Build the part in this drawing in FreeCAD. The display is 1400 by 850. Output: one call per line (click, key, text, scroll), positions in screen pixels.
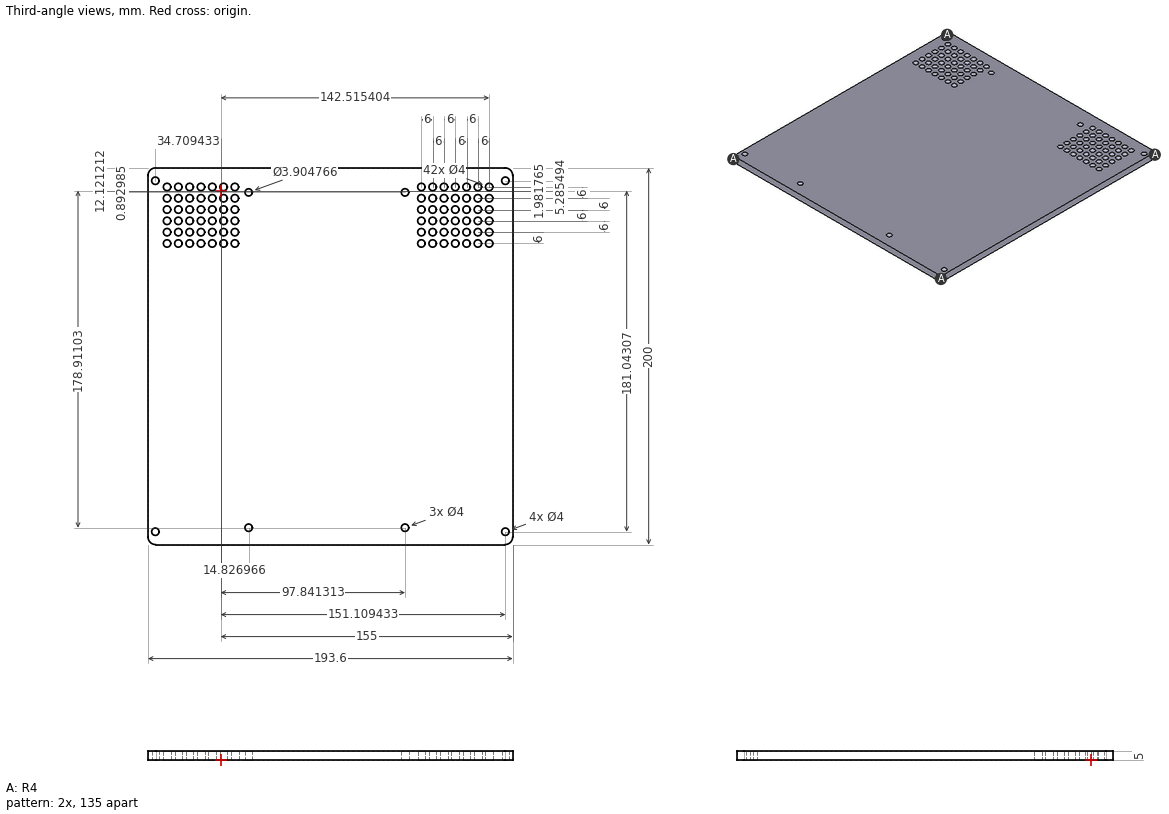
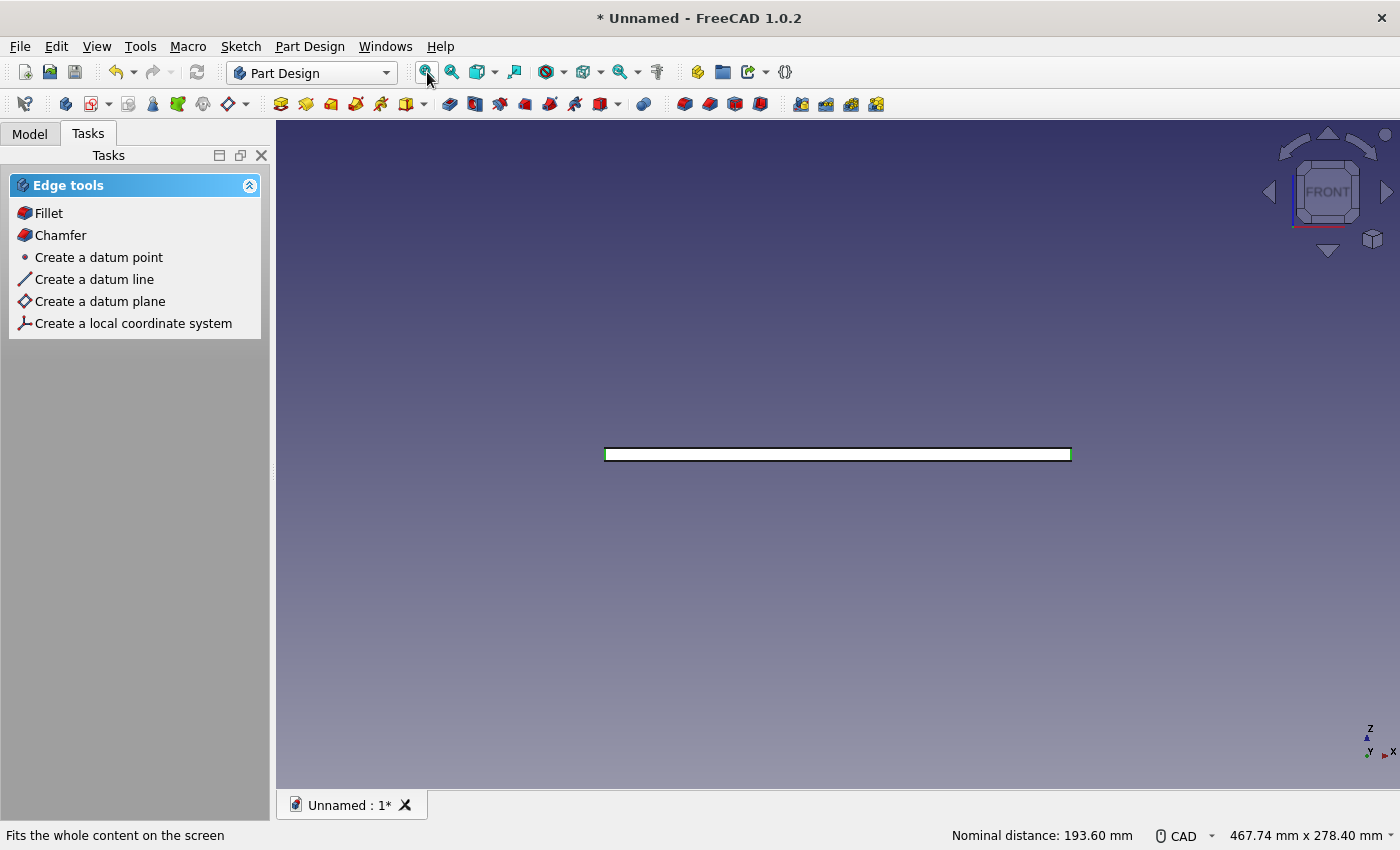
key(3)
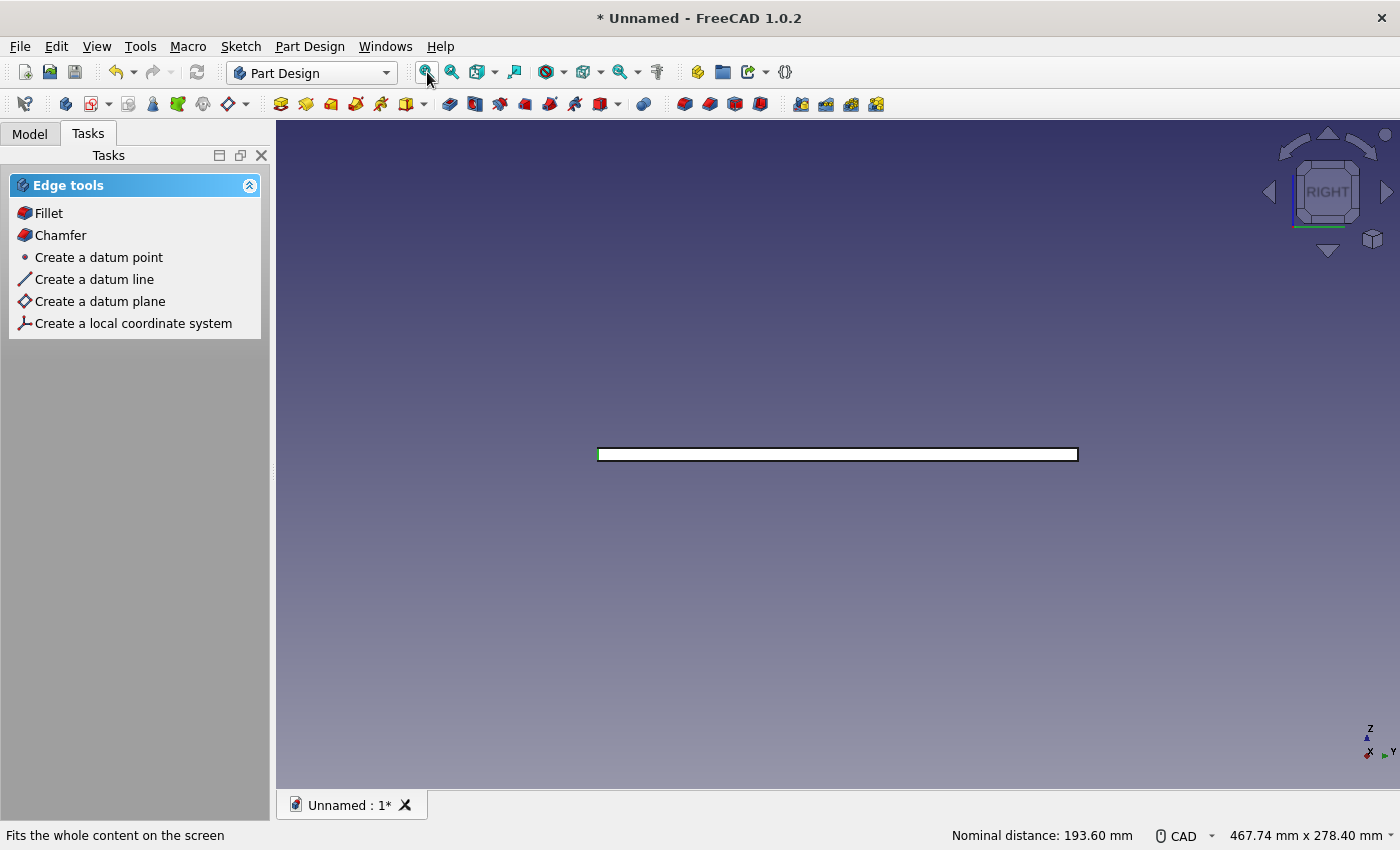
click(427, 72)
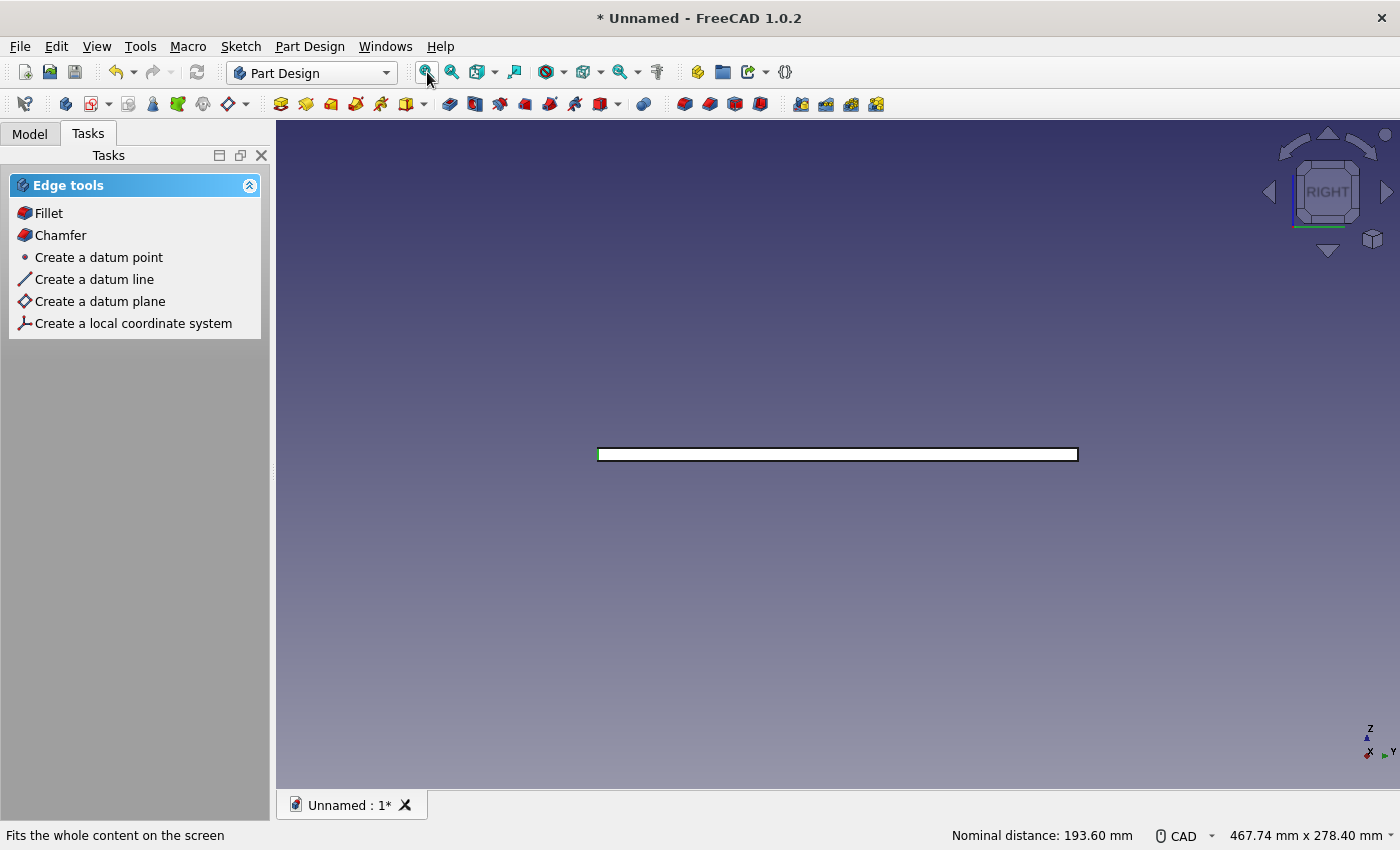
scroll(1078, 453, up, 7)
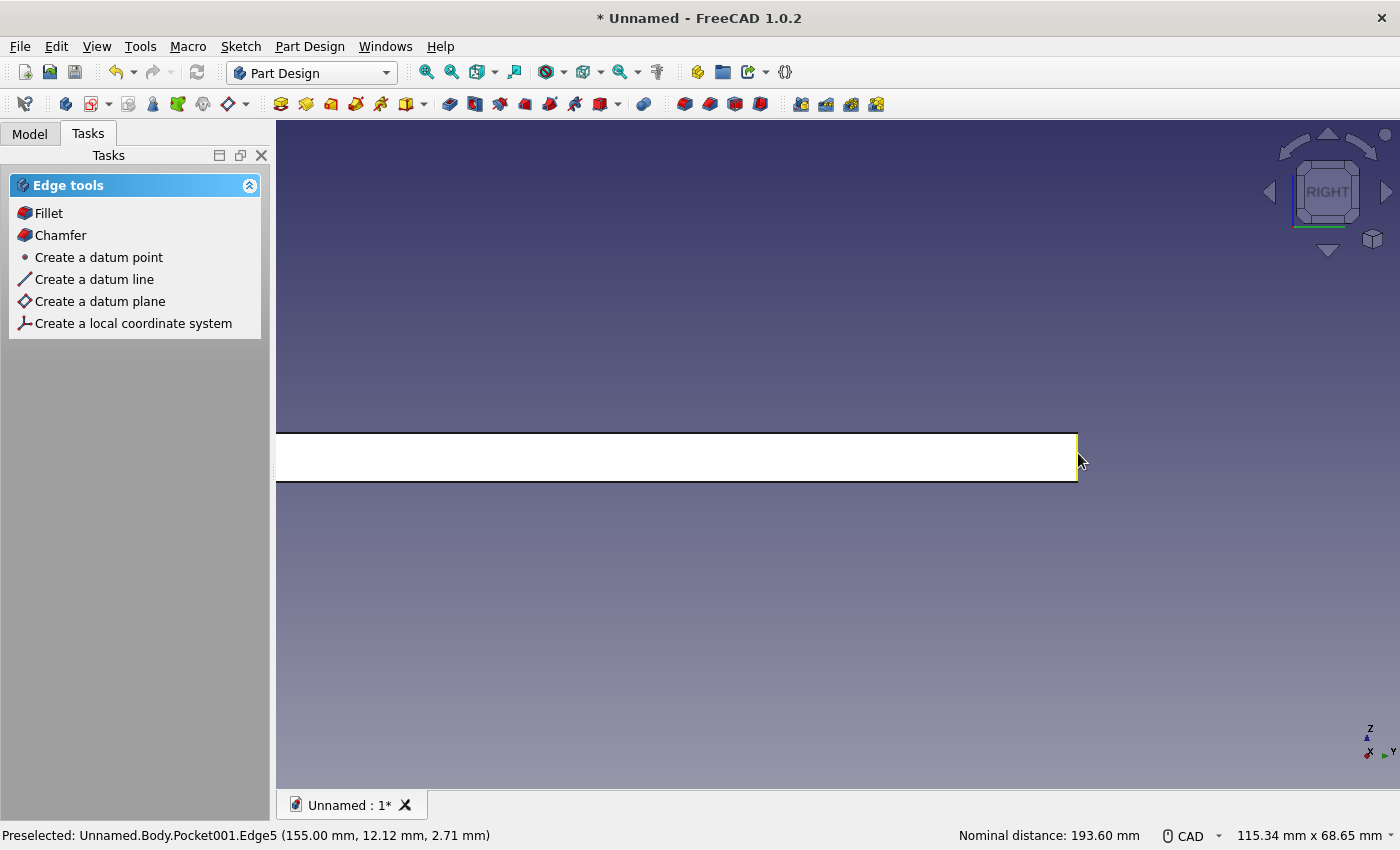
click(1077, 457, ctrl)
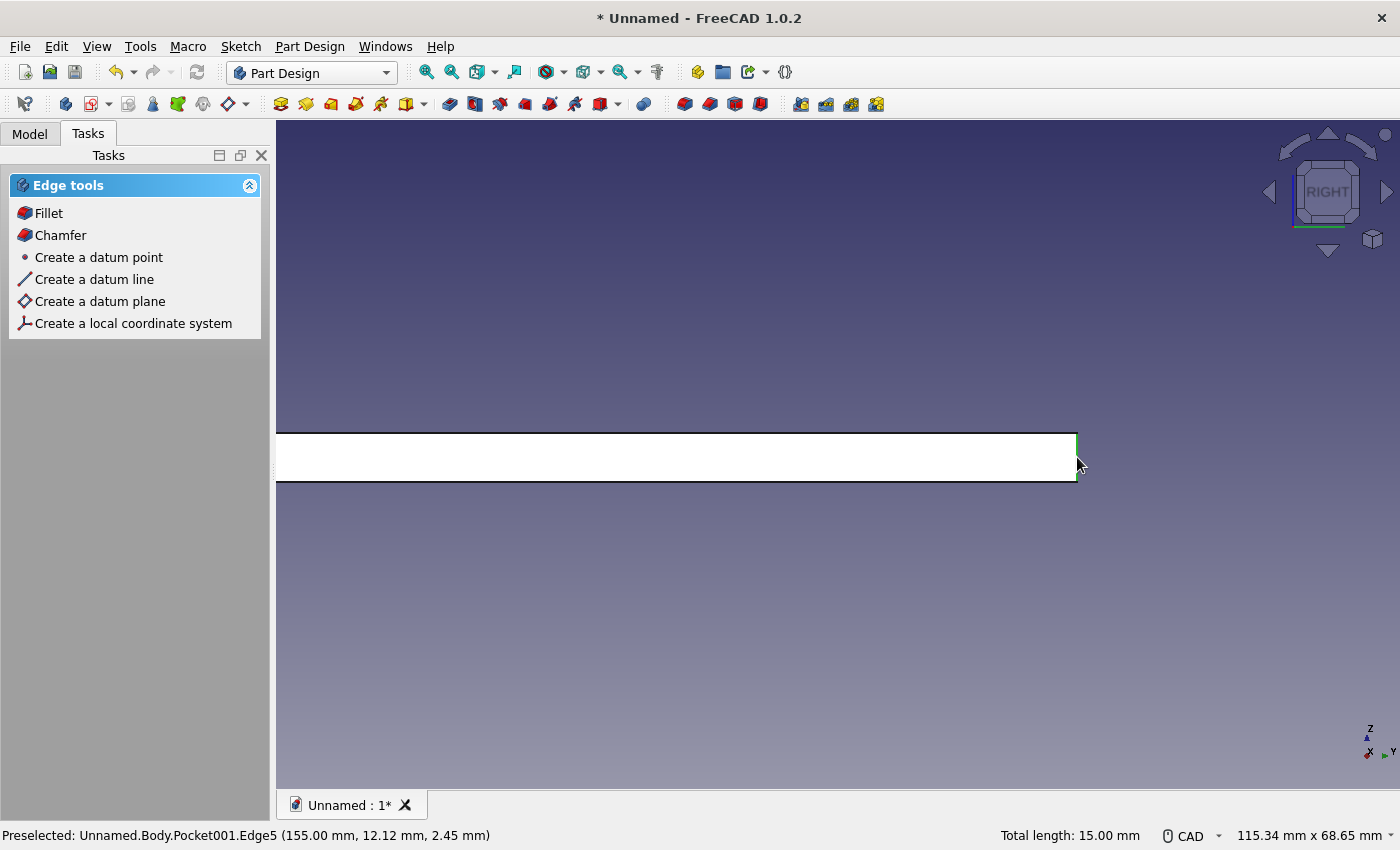
click(427, 72)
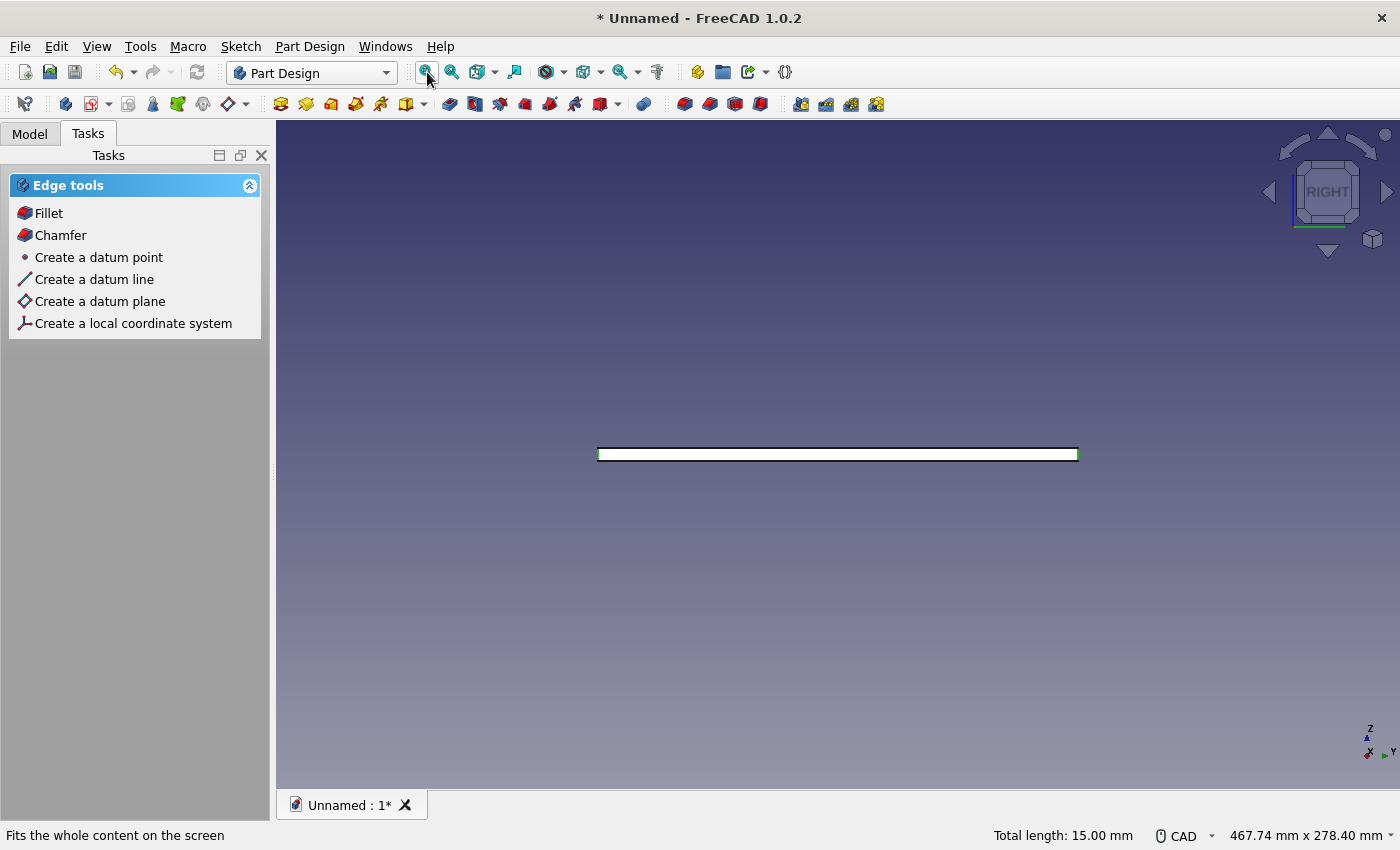
key(5)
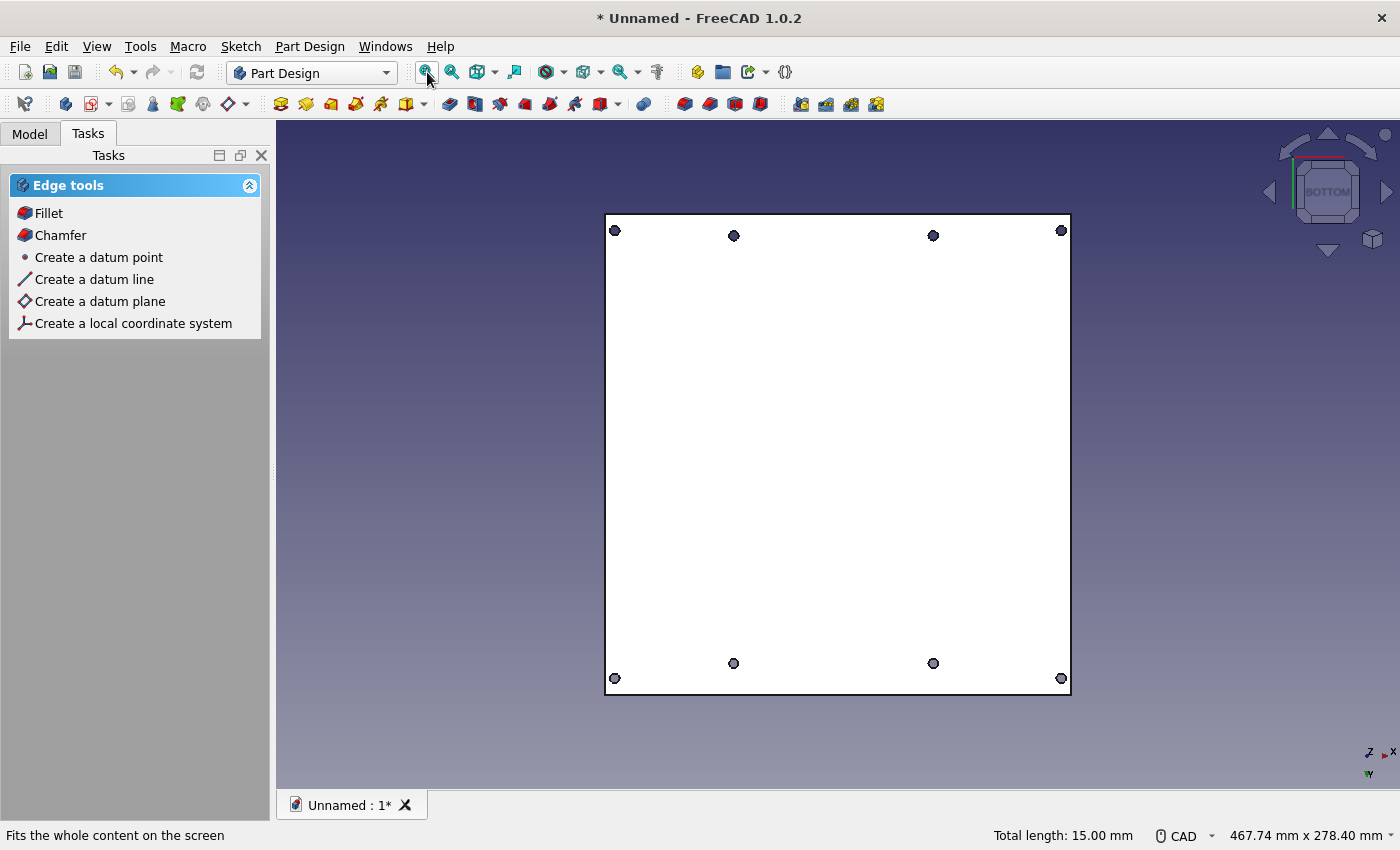
scroll(605, 694, up, 7)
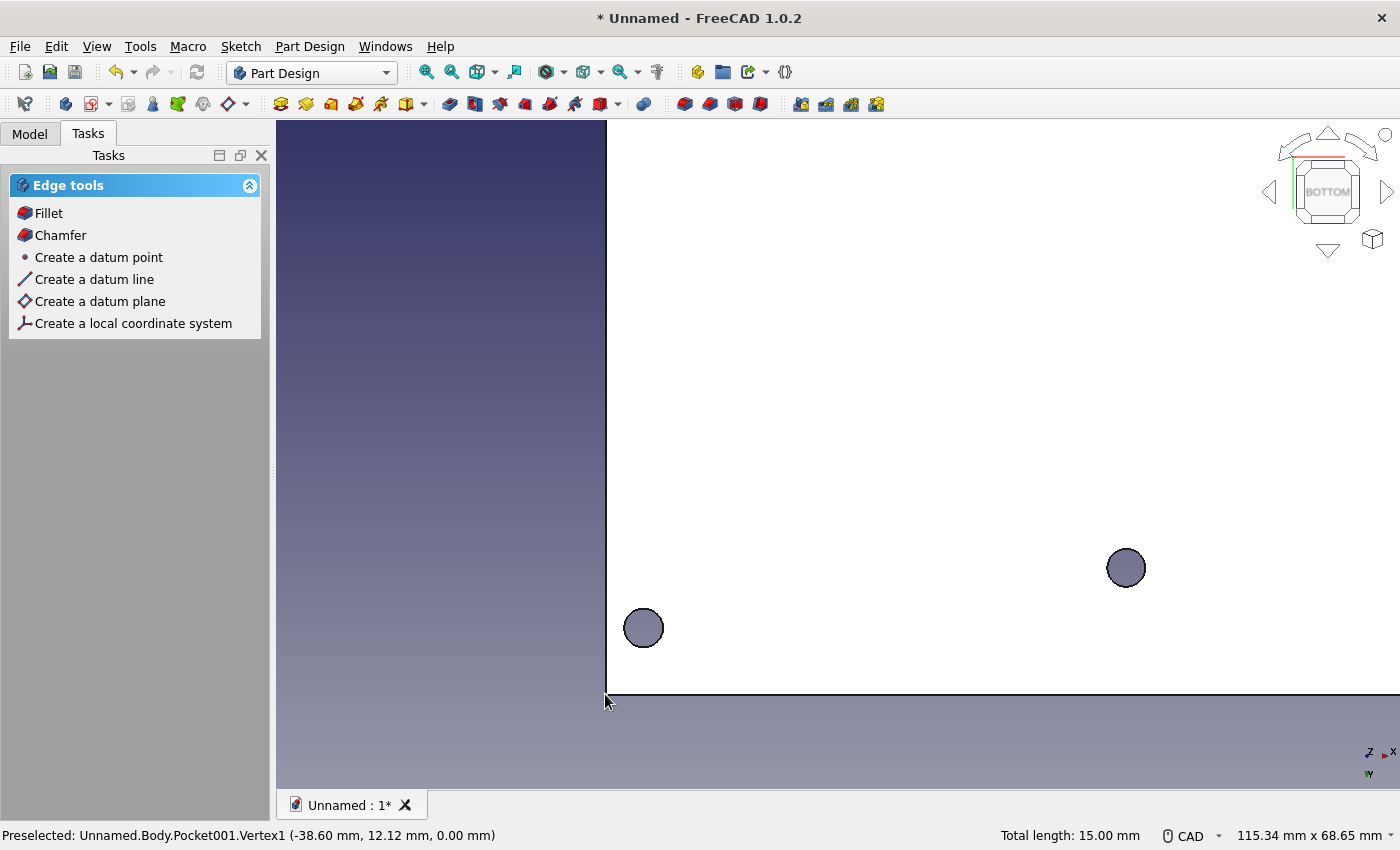
click(427, 72)